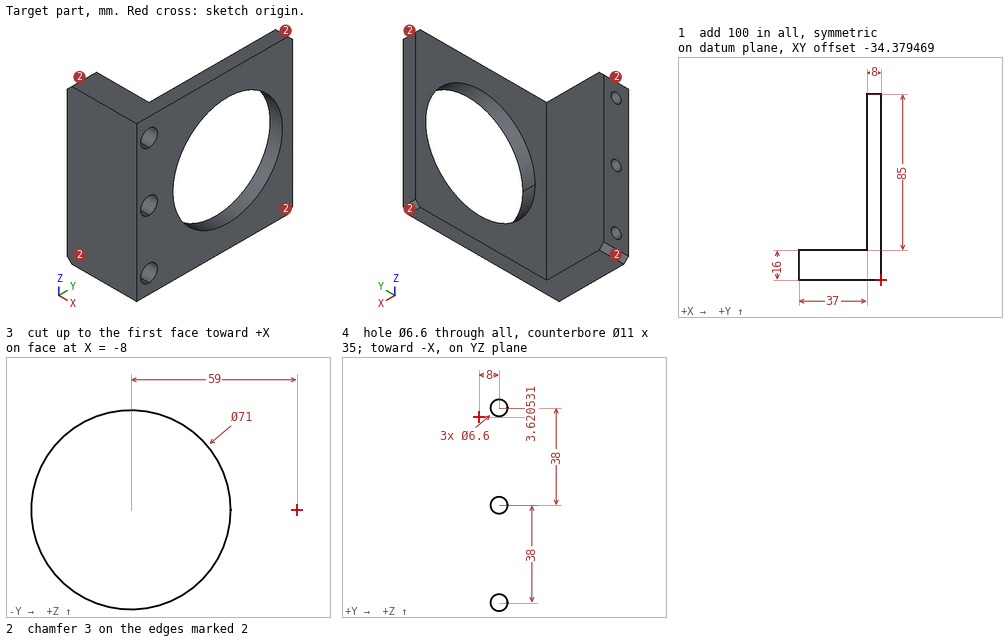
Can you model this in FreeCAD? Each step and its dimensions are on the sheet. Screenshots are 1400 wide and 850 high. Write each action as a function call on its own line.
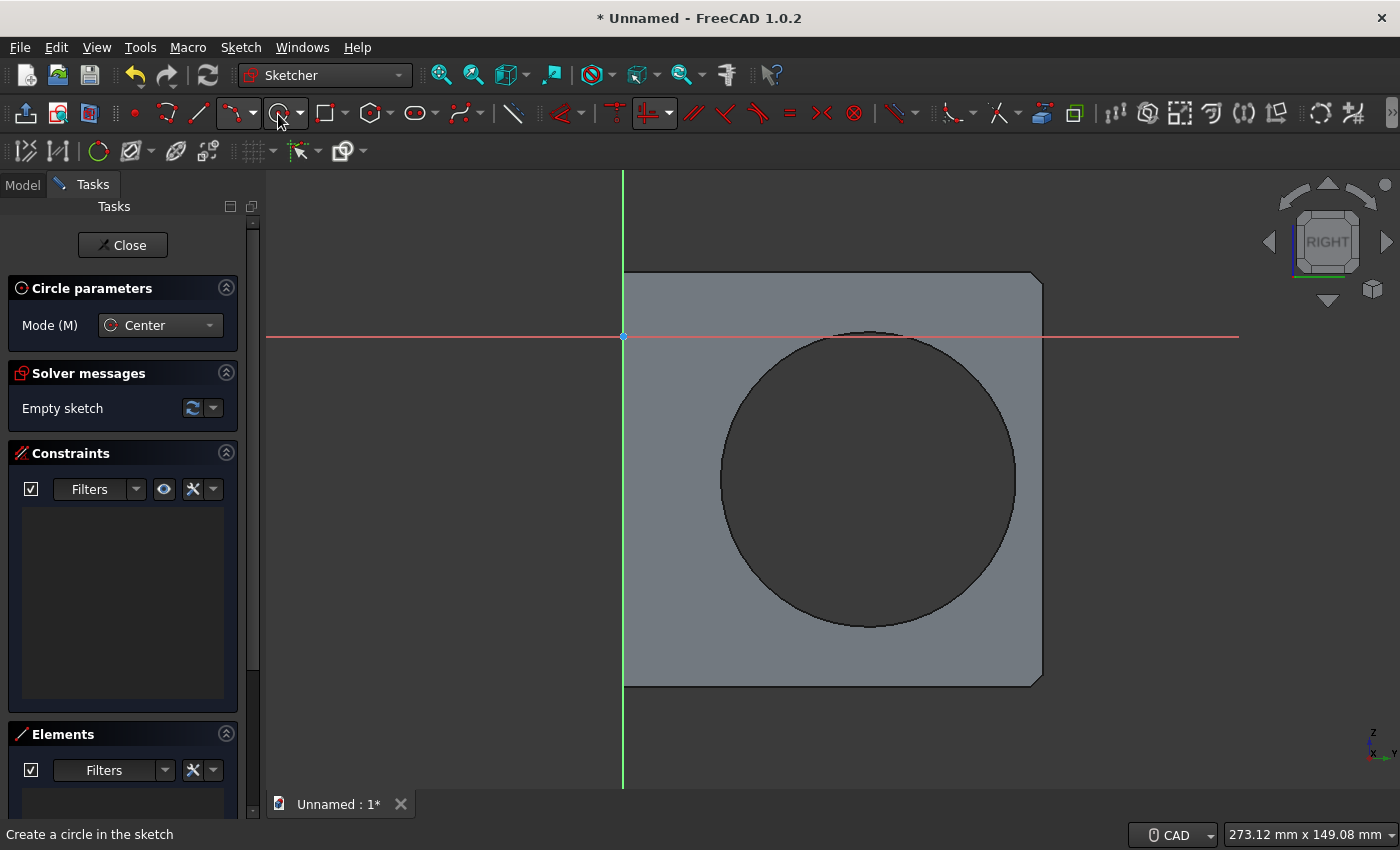
scroll(657, 322, up, 3)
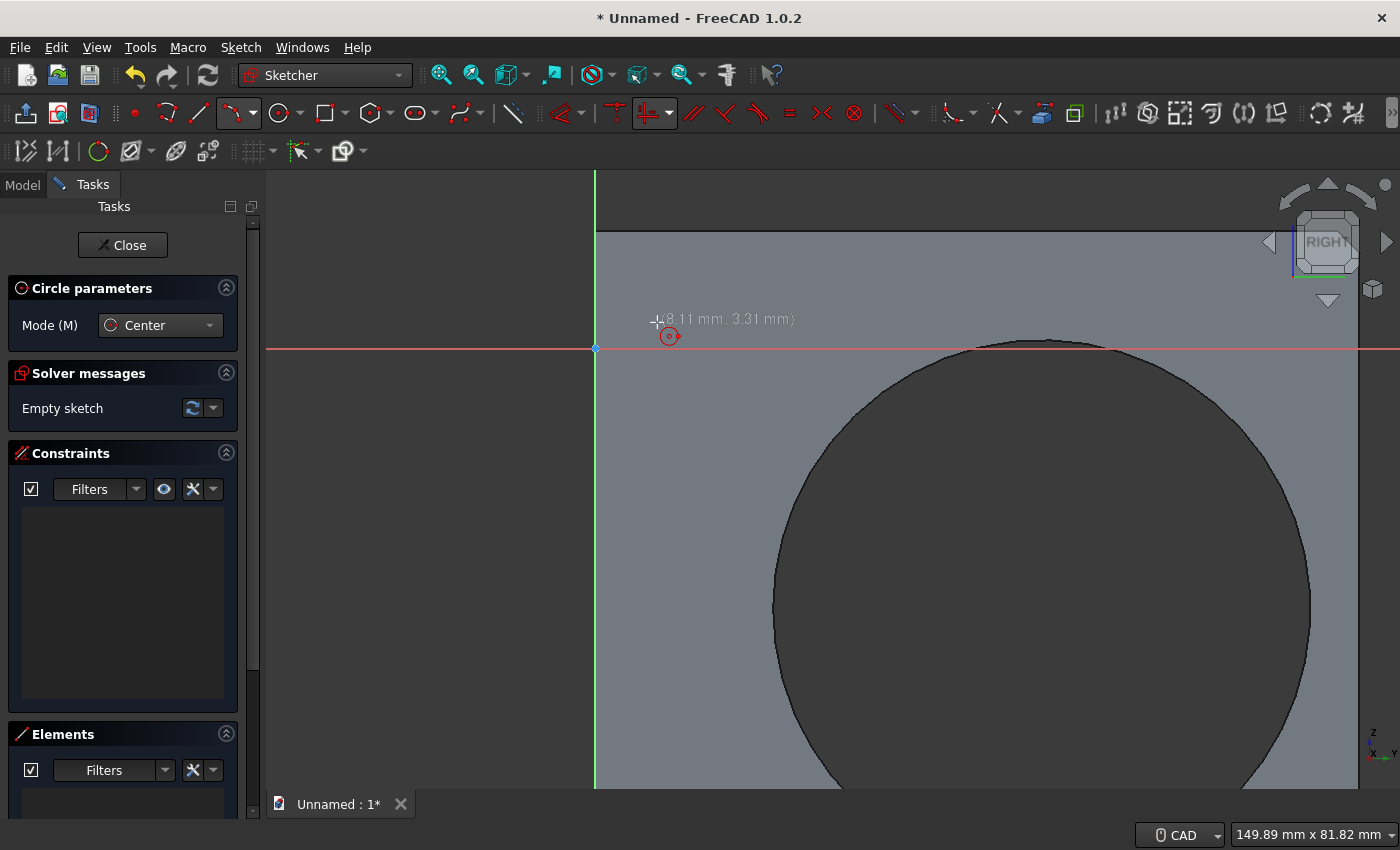
click(656, 321)
click(674, 304)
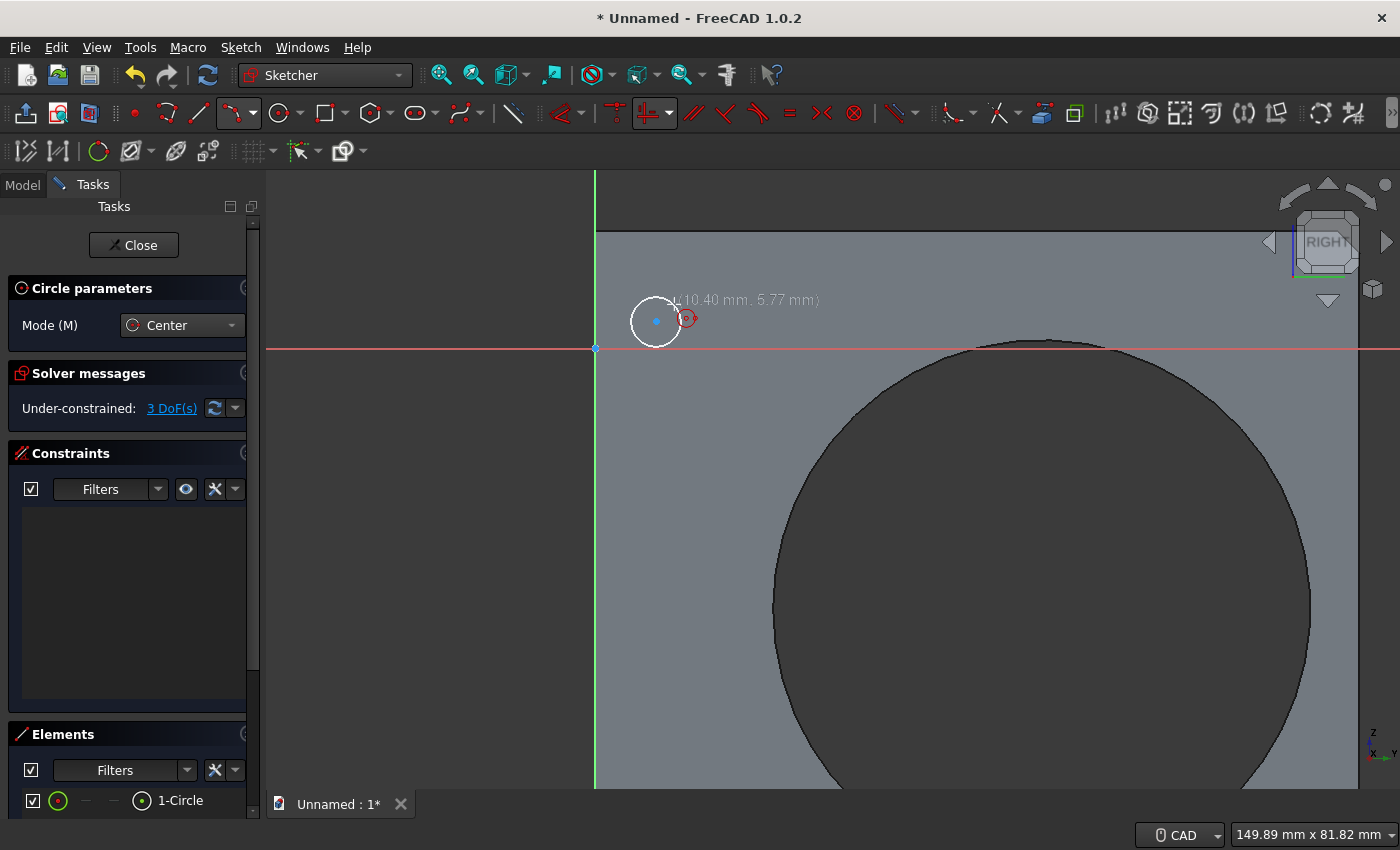
click(656, 609)
click(674, 591)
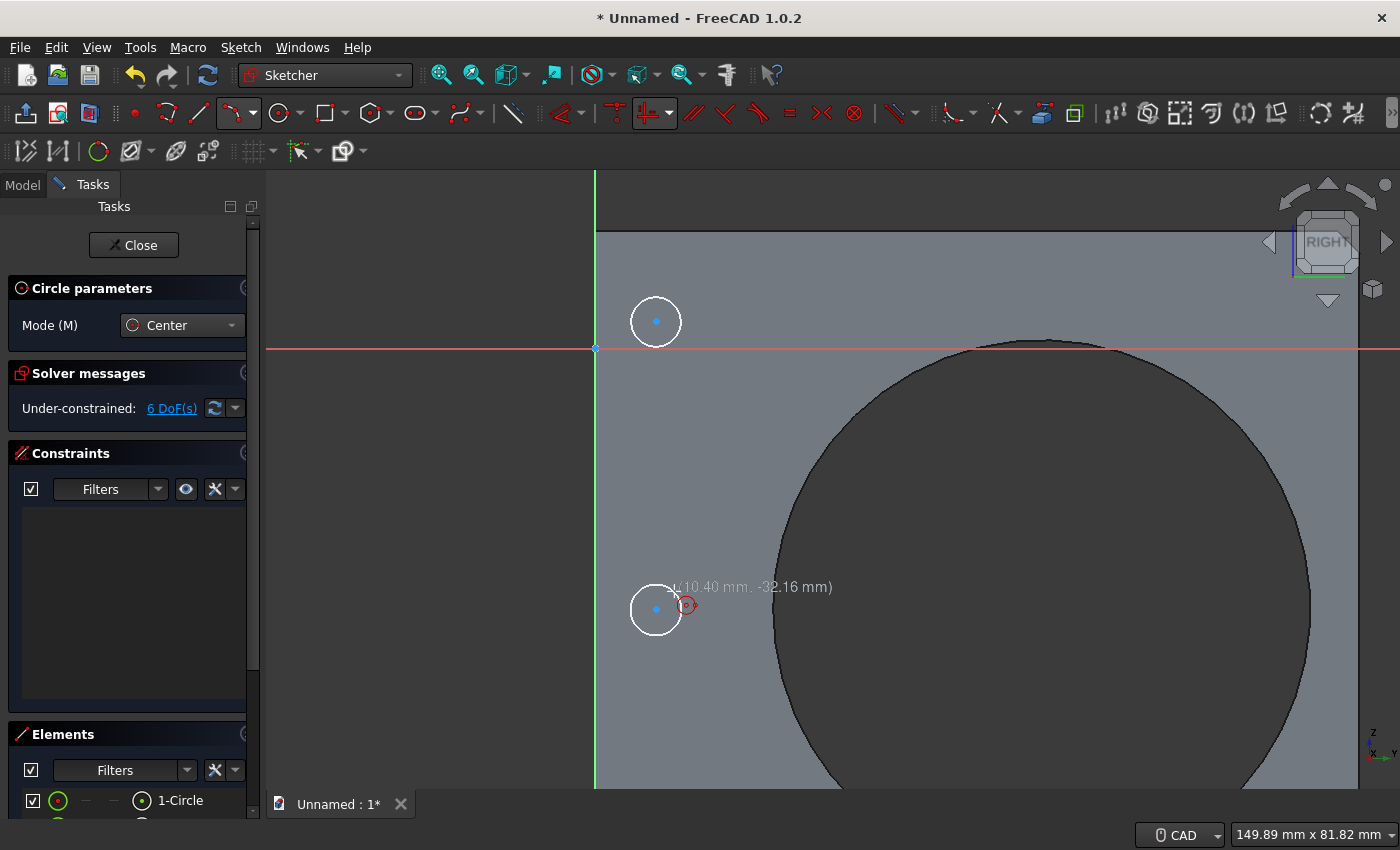
scroll(1022, 217, down, 2)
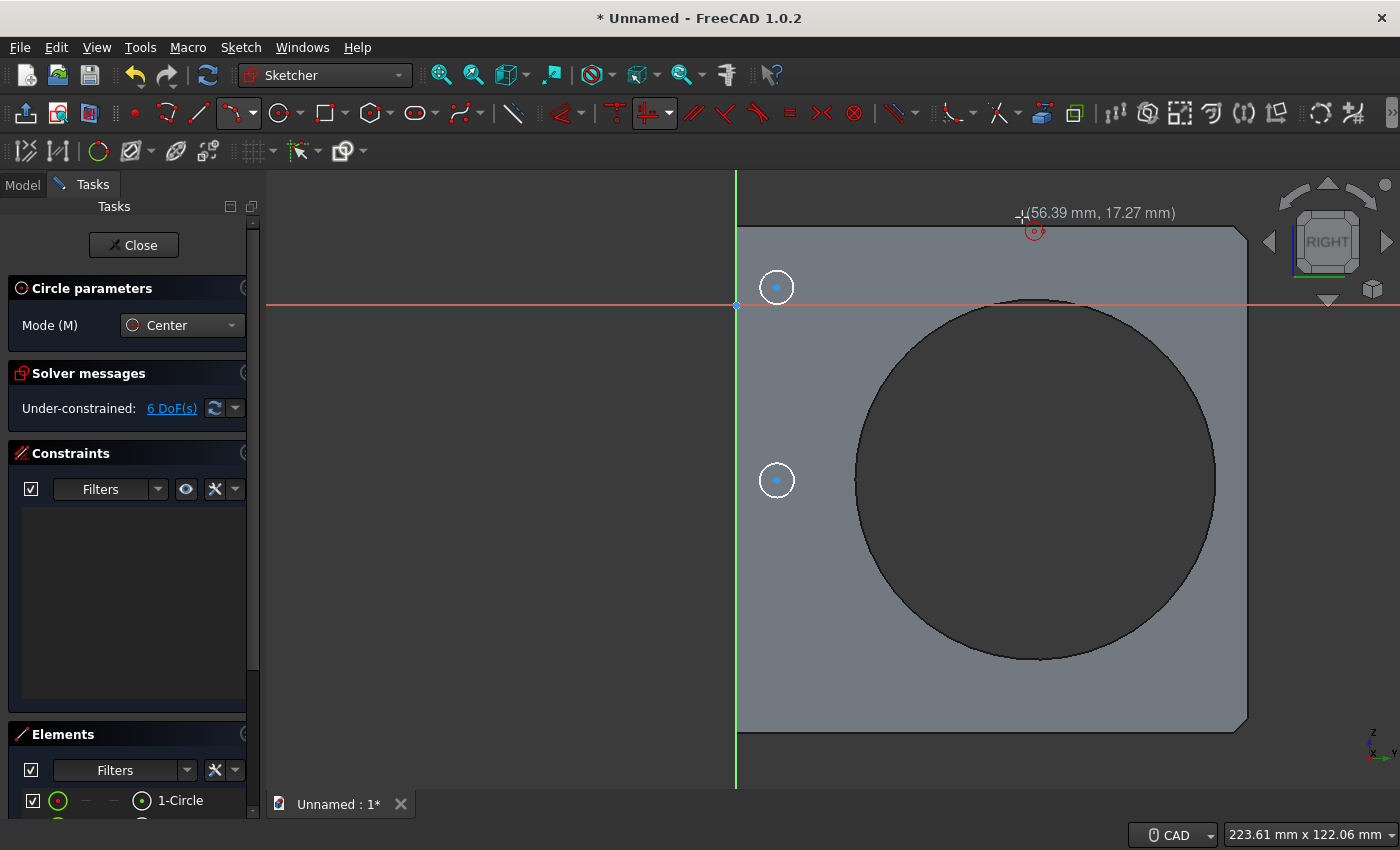
scroll(777, 672, up, 2)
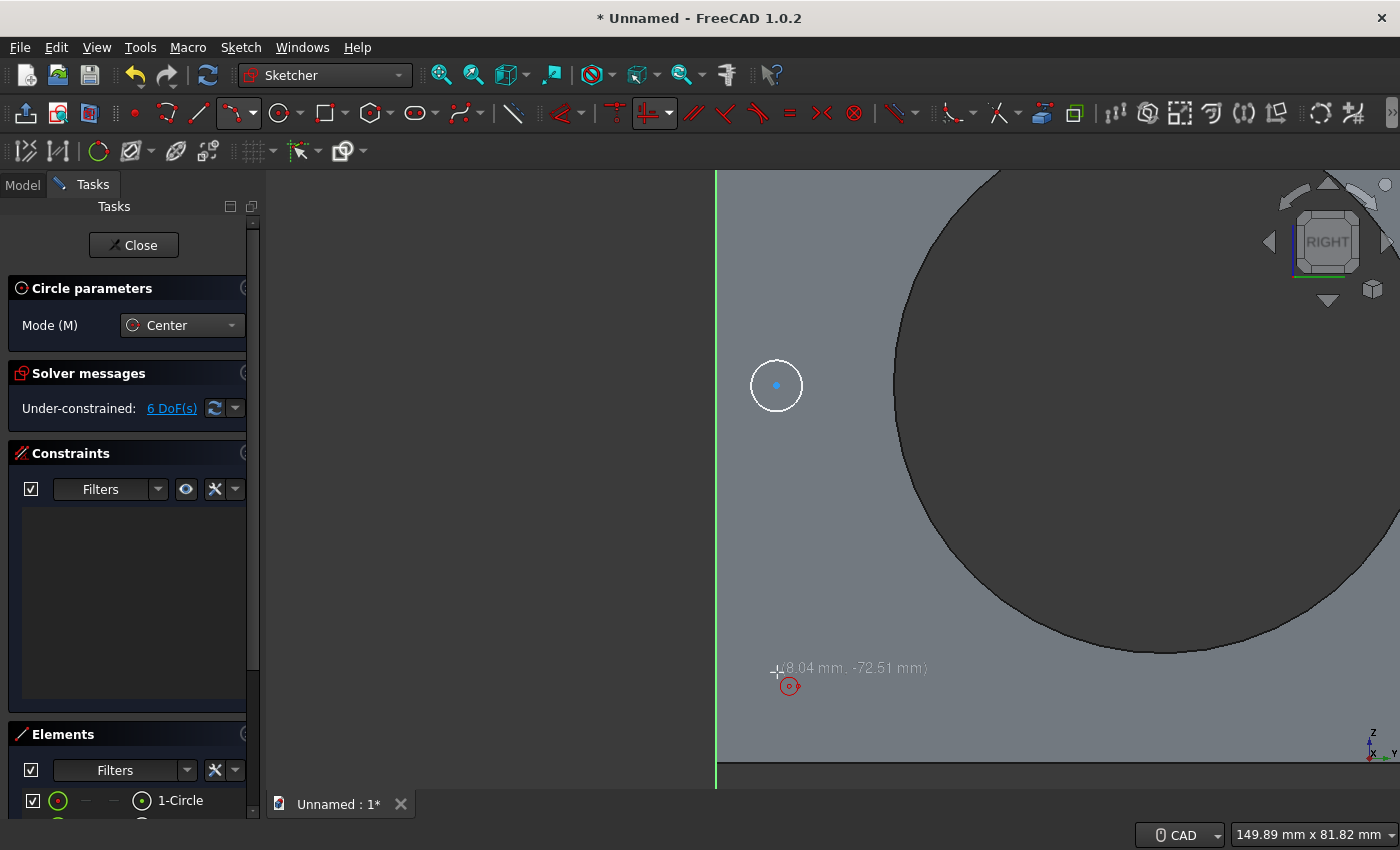
click(776, 672)
click(794, 654)
key(Escape)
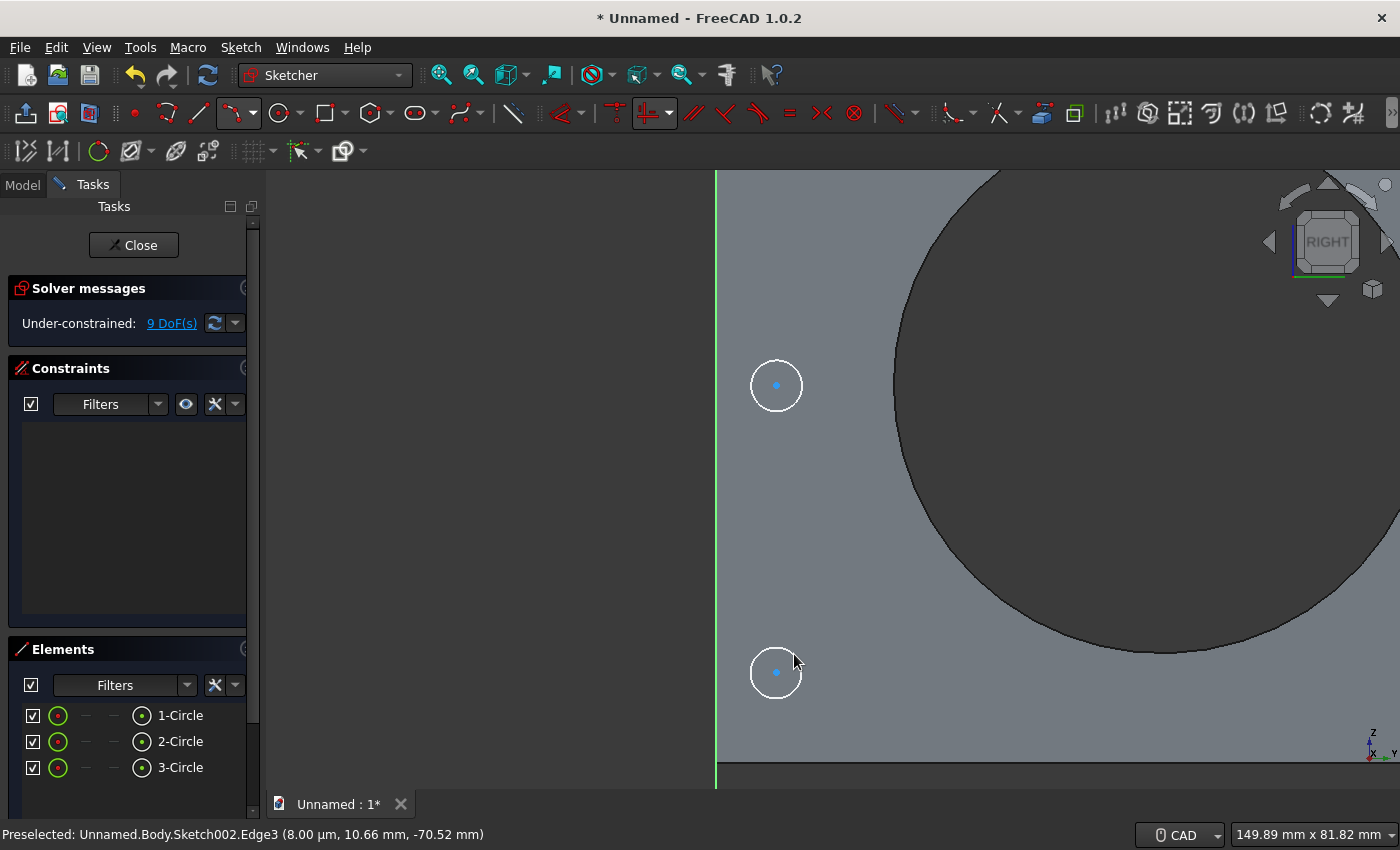
scroll(776, 672, down, 2)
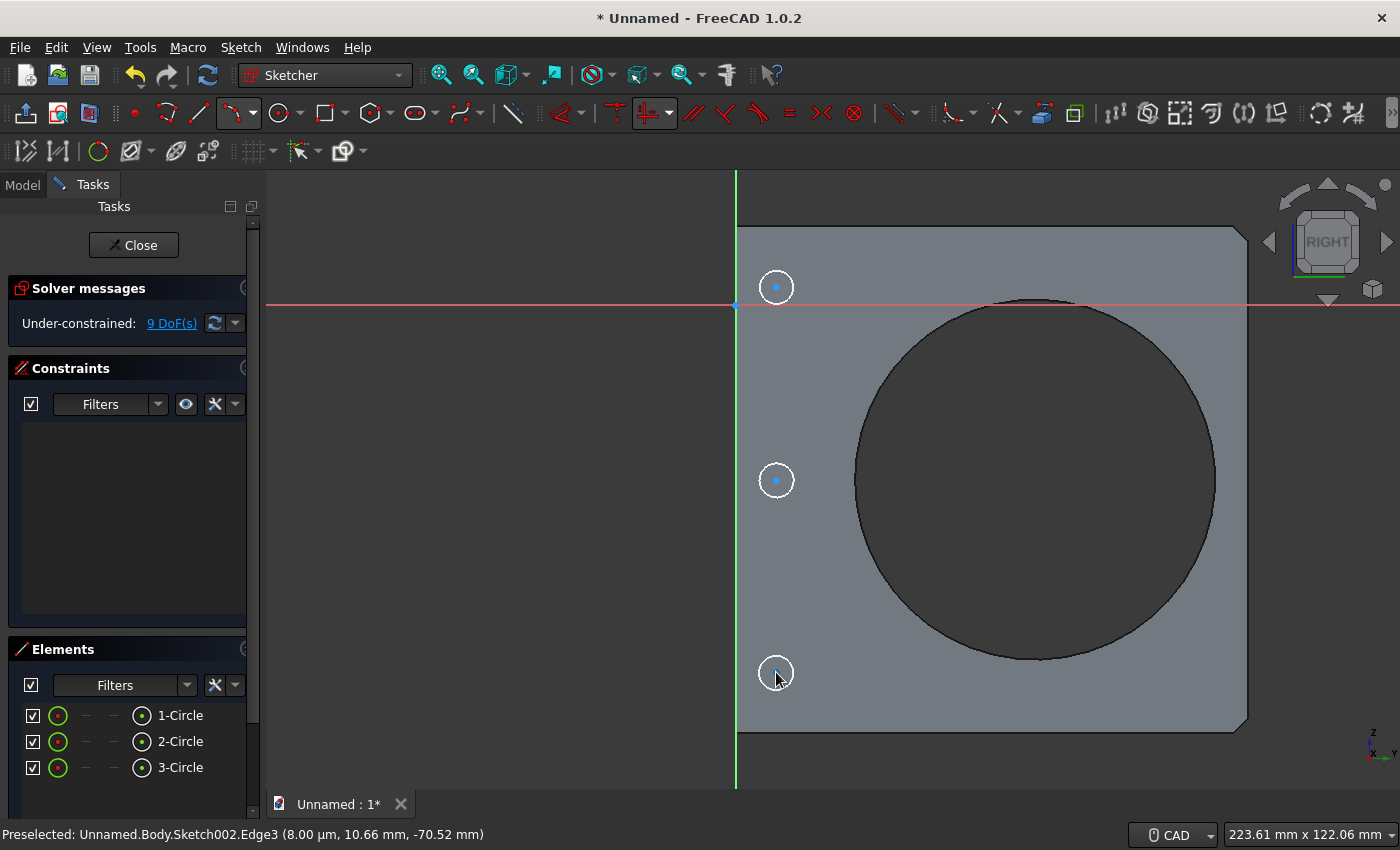
click(788, 276)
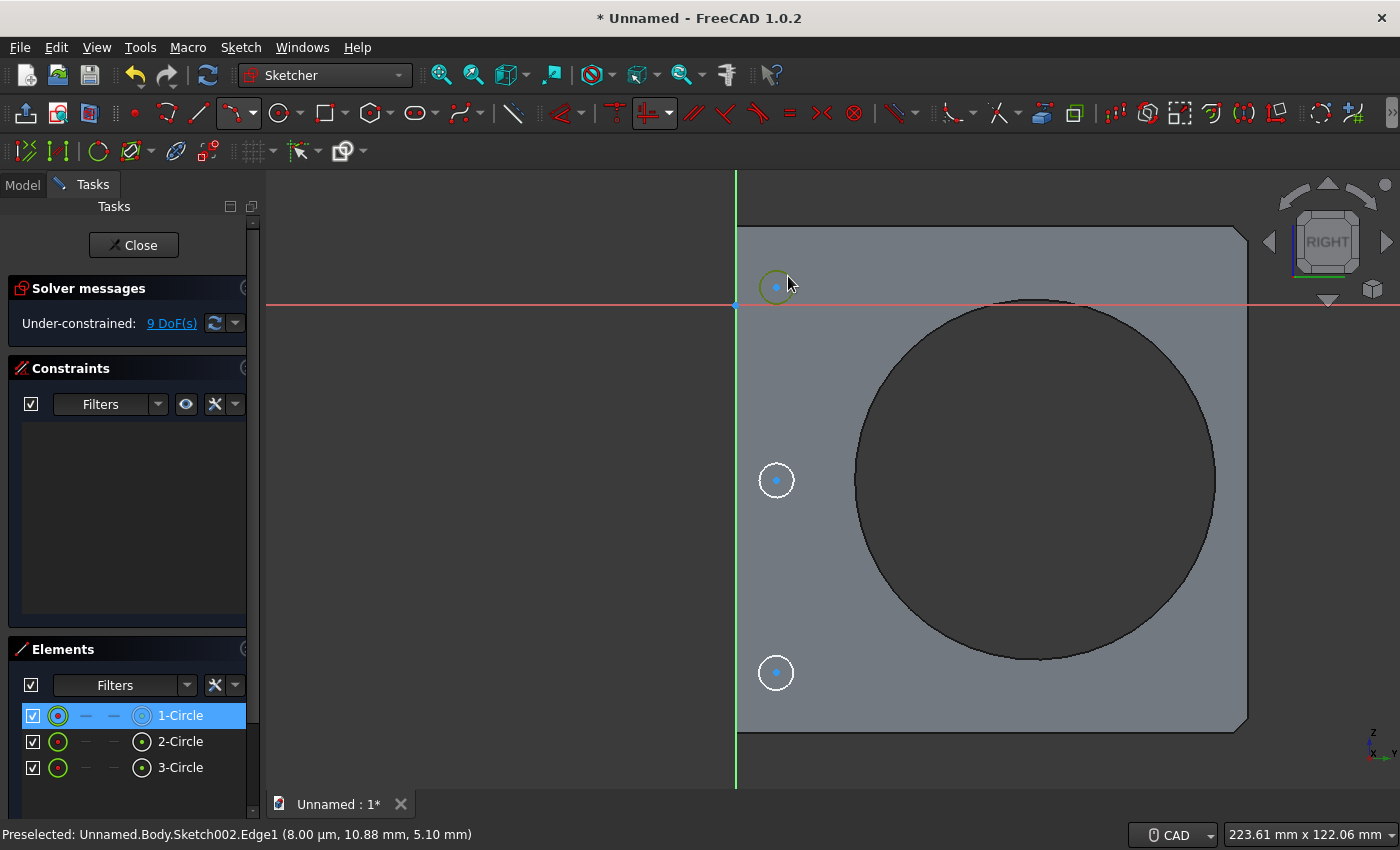
click(789, 468)